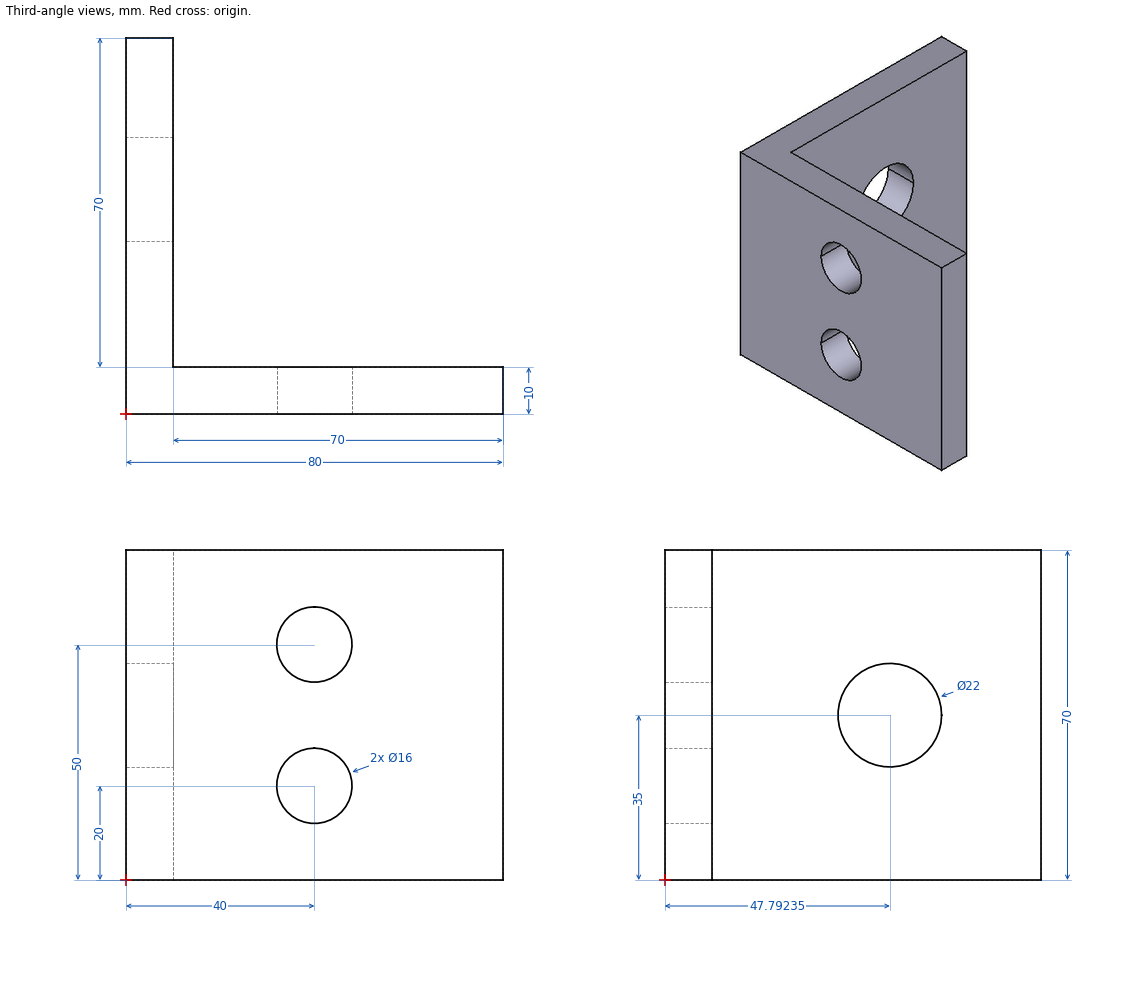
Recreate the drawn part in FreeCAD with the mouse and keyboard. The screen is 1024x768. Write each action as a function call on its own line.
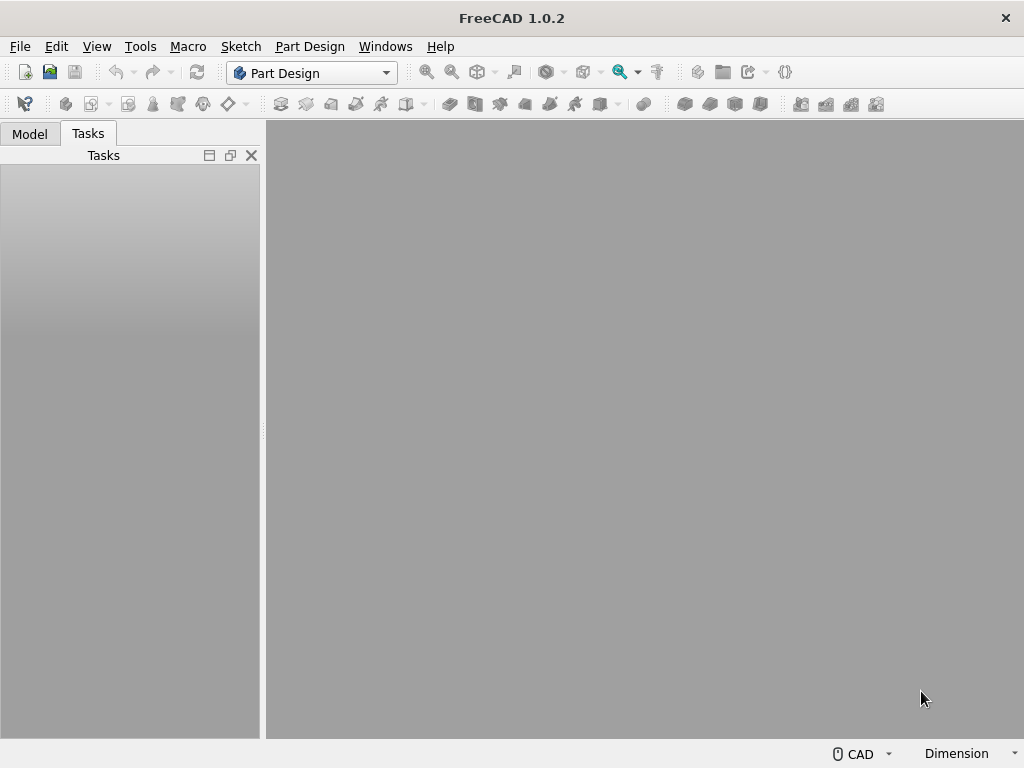
click(25, 72)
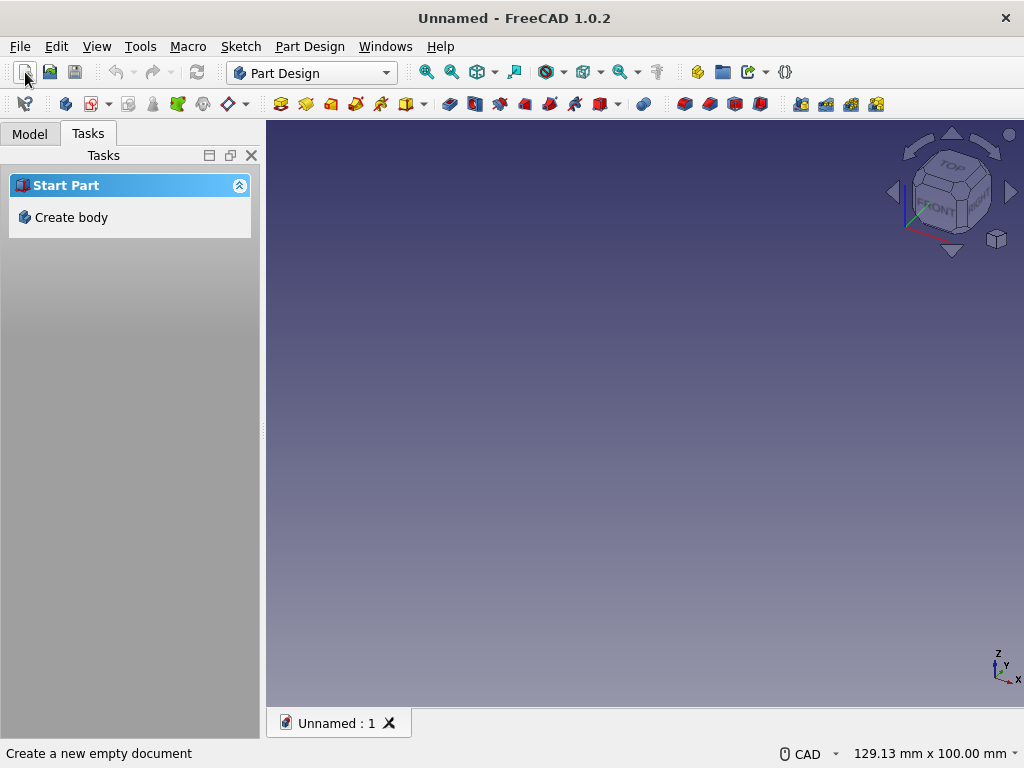
click(90, 104)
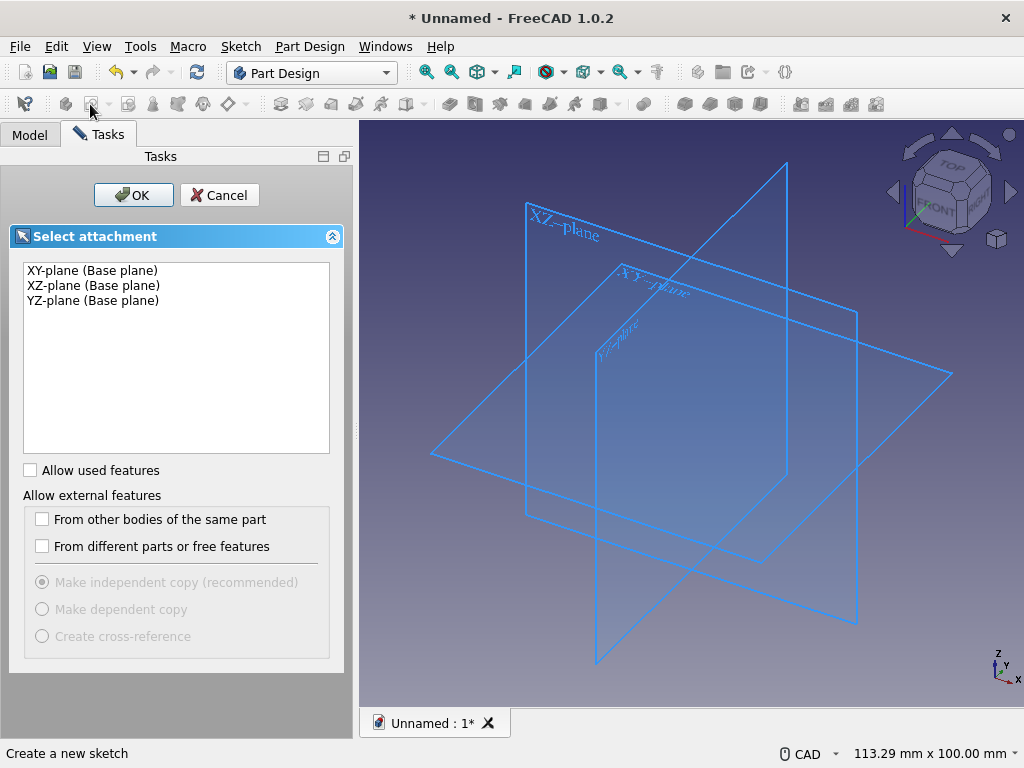
click(84, 270)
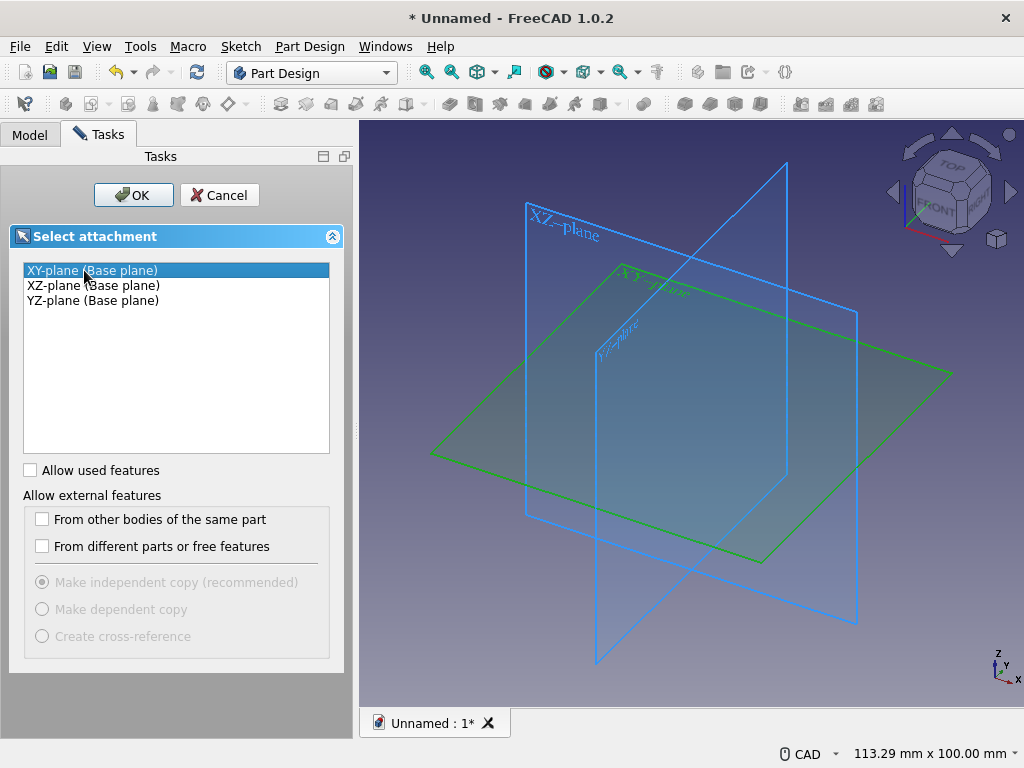
click(134, 195)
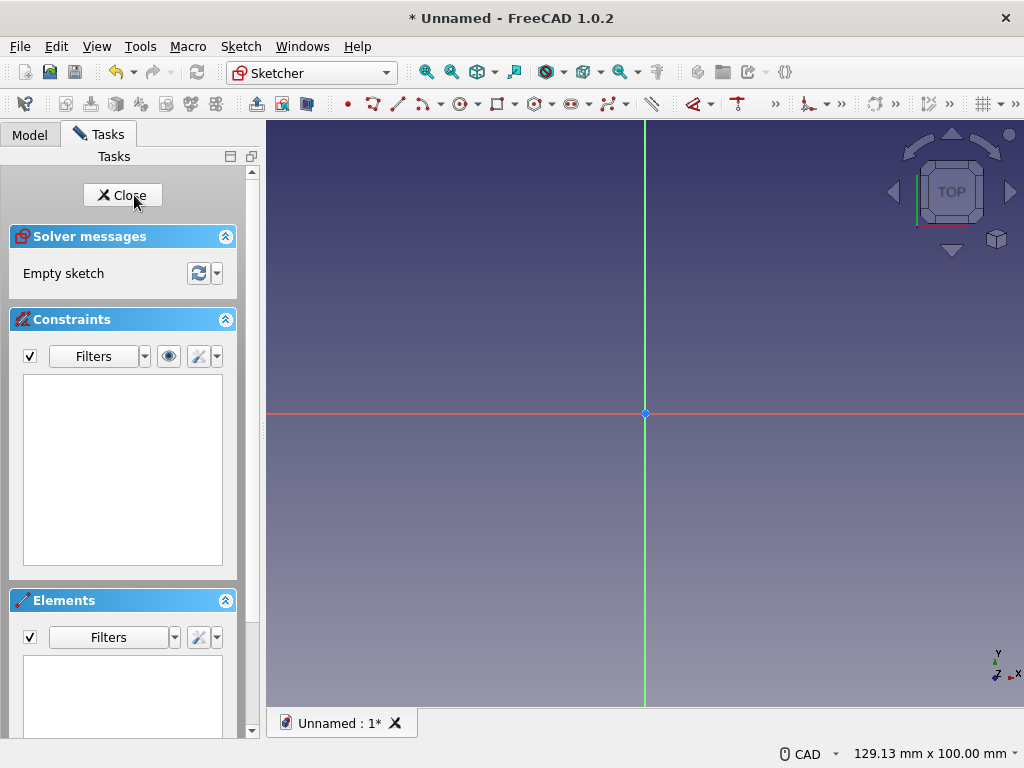
scroll(294, 679, down, 3)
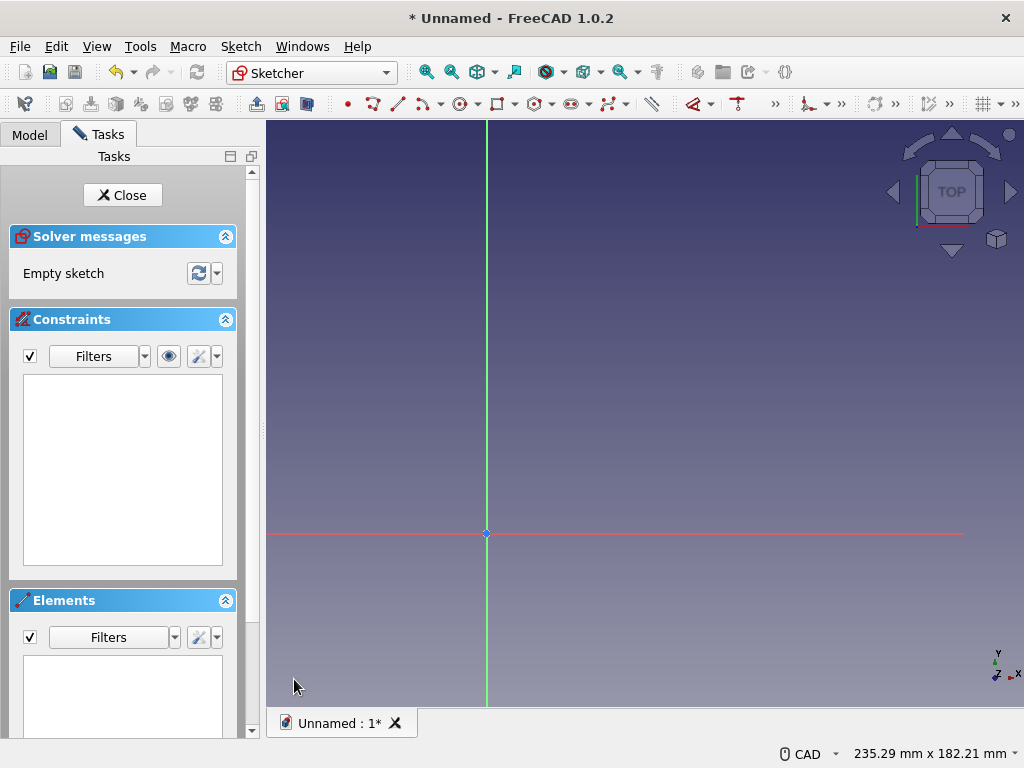
scroll(695, 387, up, 2)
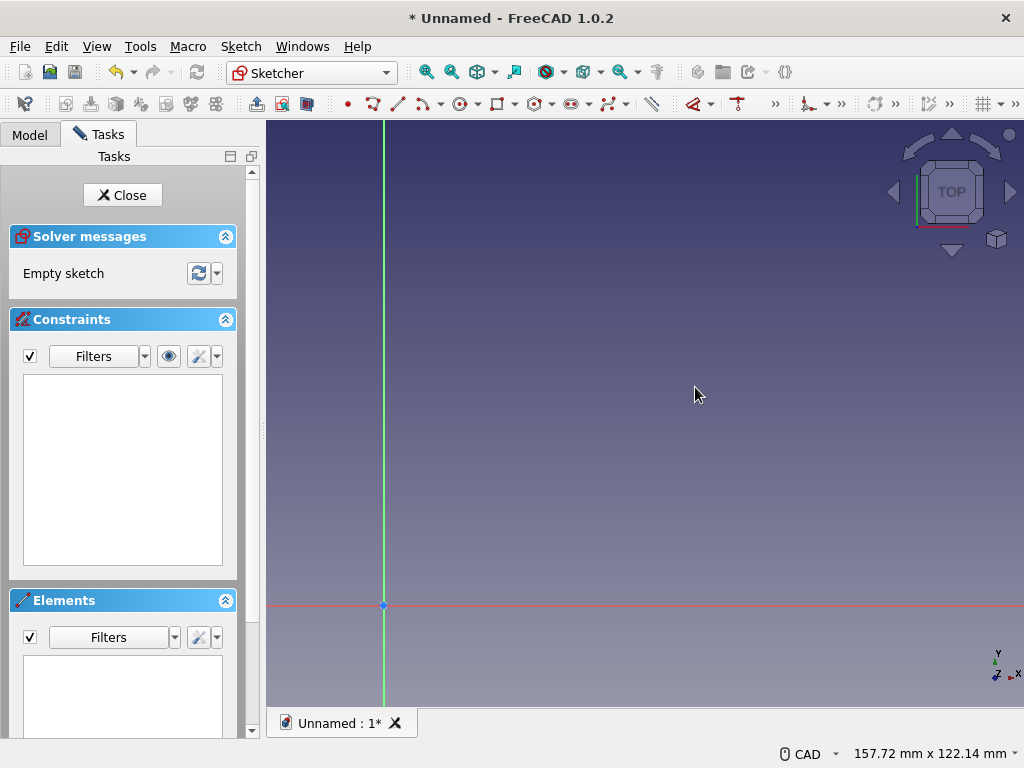
click(373, 104)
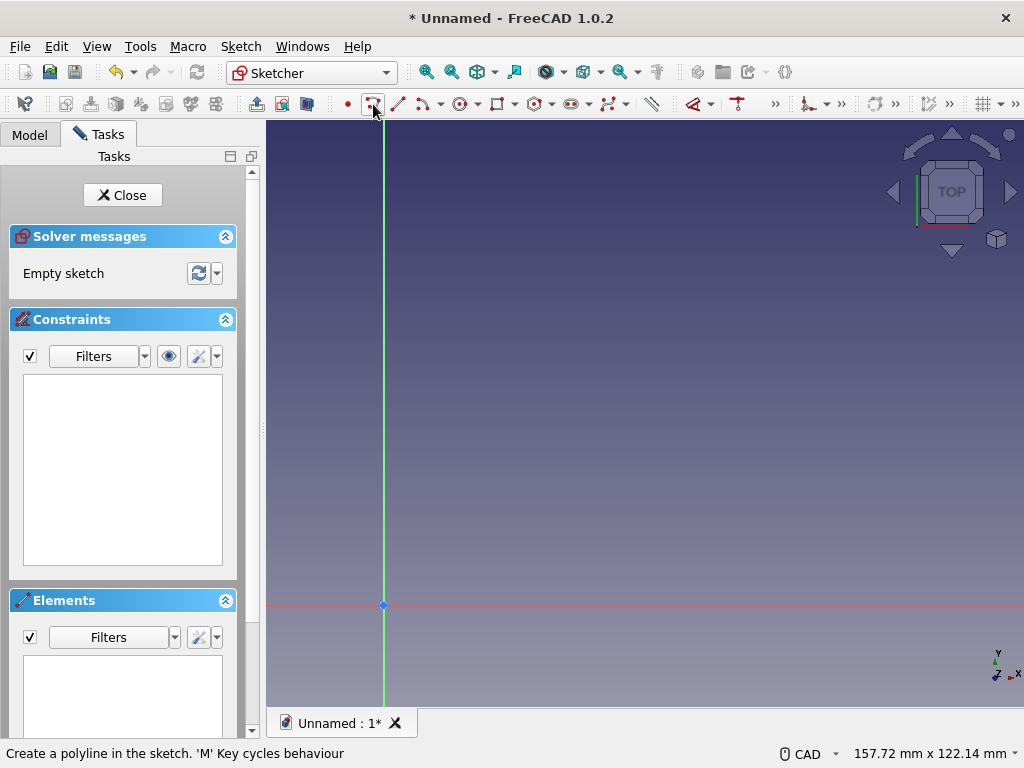
click(384, 606)
click(768, 597)
click(768, 558)
click(432, 558)
click(432, 221)
click(393, 221)
click(384, 606)
key(Escape)
key(Escape)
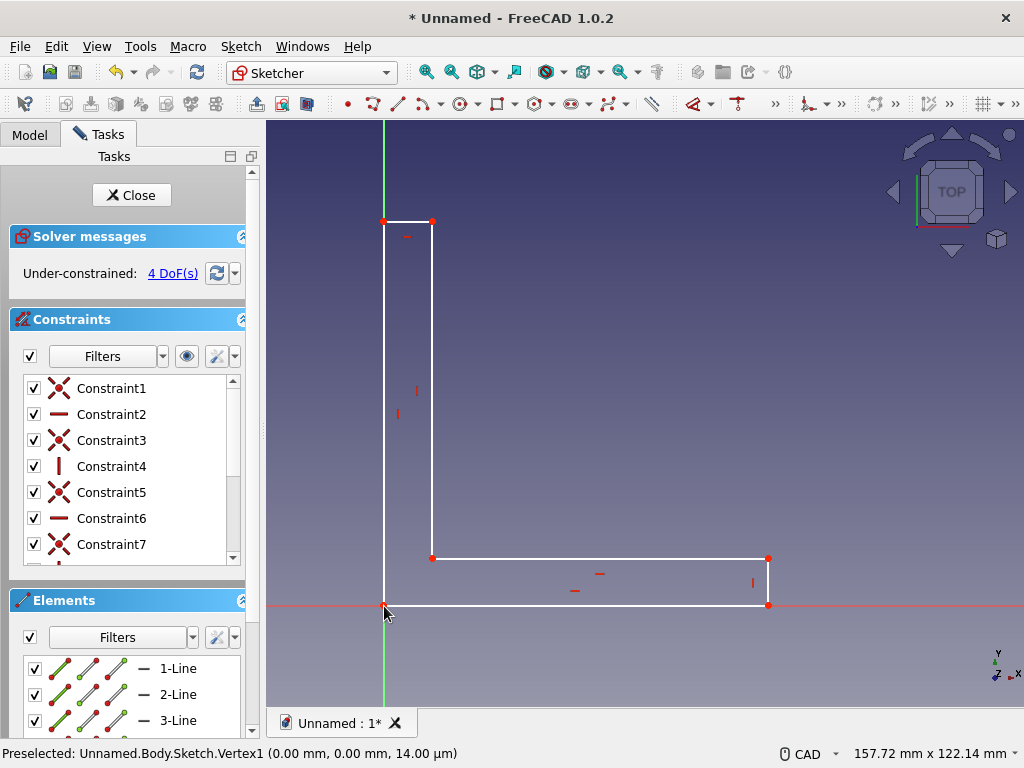
click(692, 104)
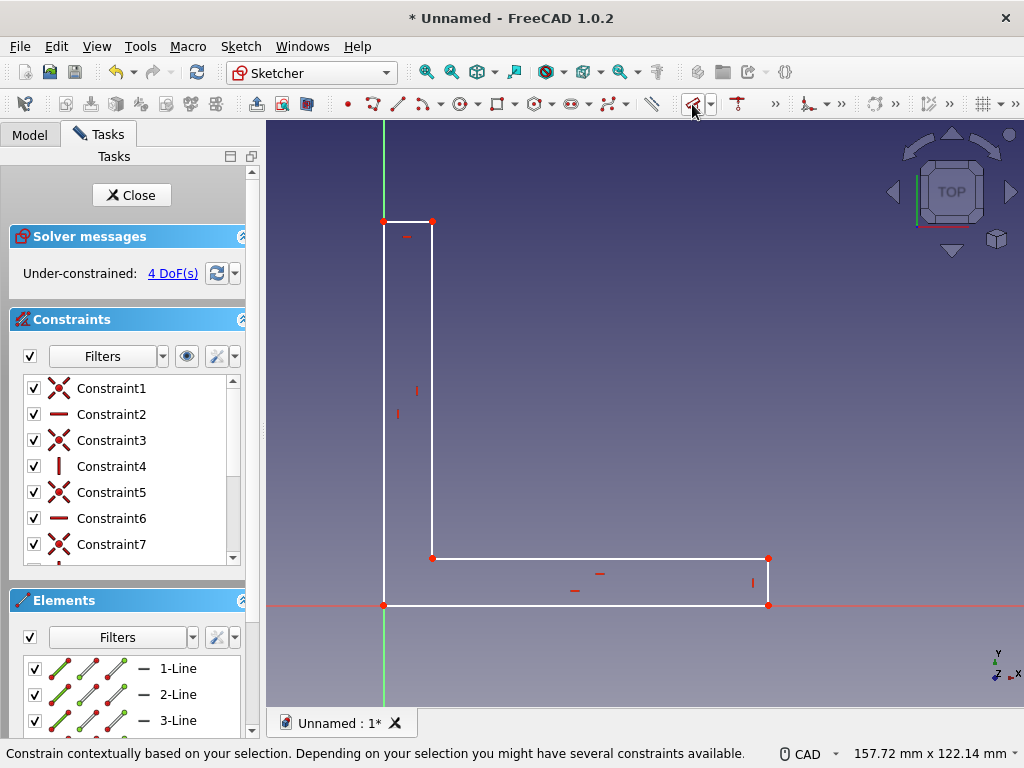
click(499, 606)
click(576, 640)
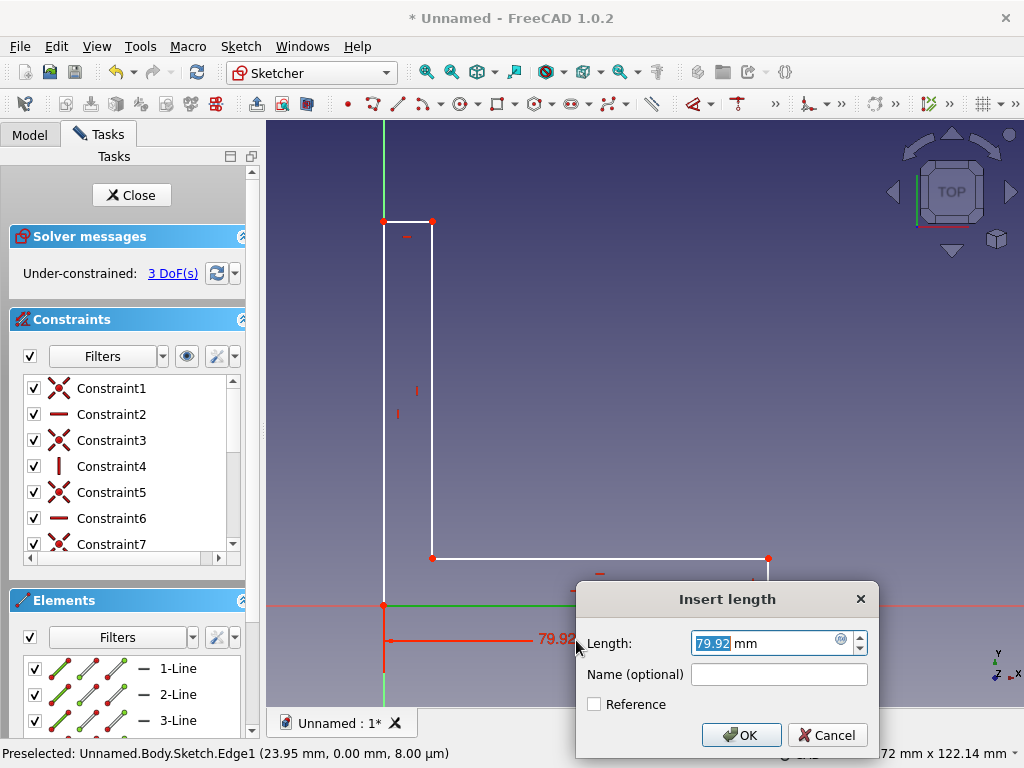
text(80)
key(Return)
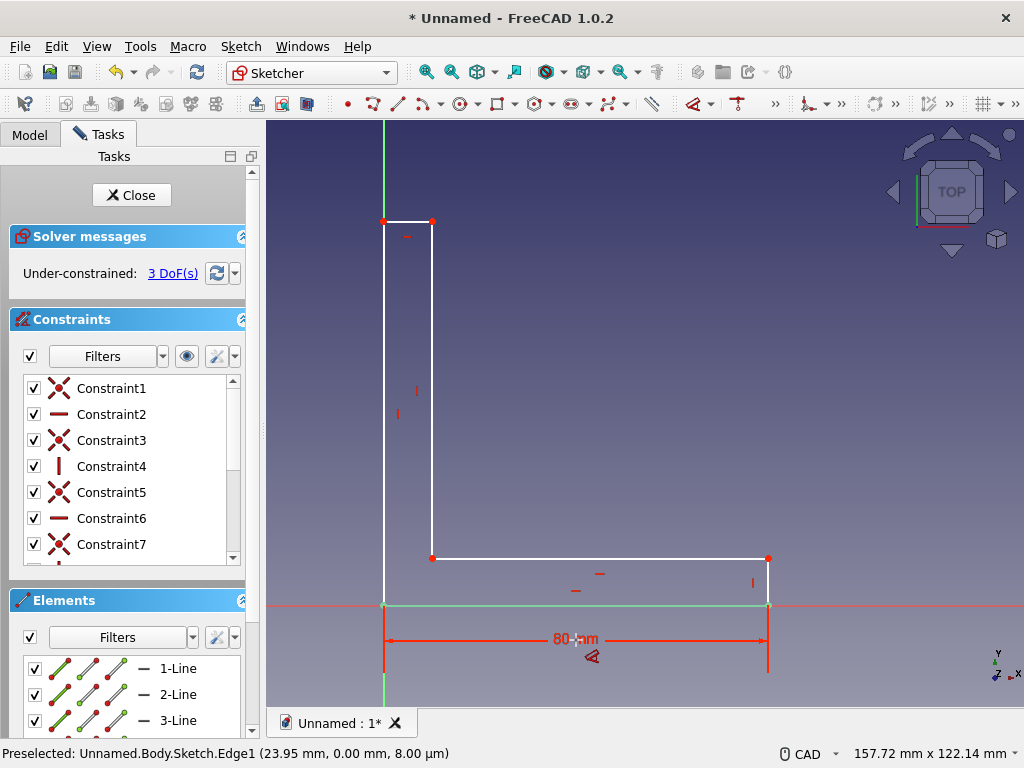
click(768, 592)
click(802, 582)